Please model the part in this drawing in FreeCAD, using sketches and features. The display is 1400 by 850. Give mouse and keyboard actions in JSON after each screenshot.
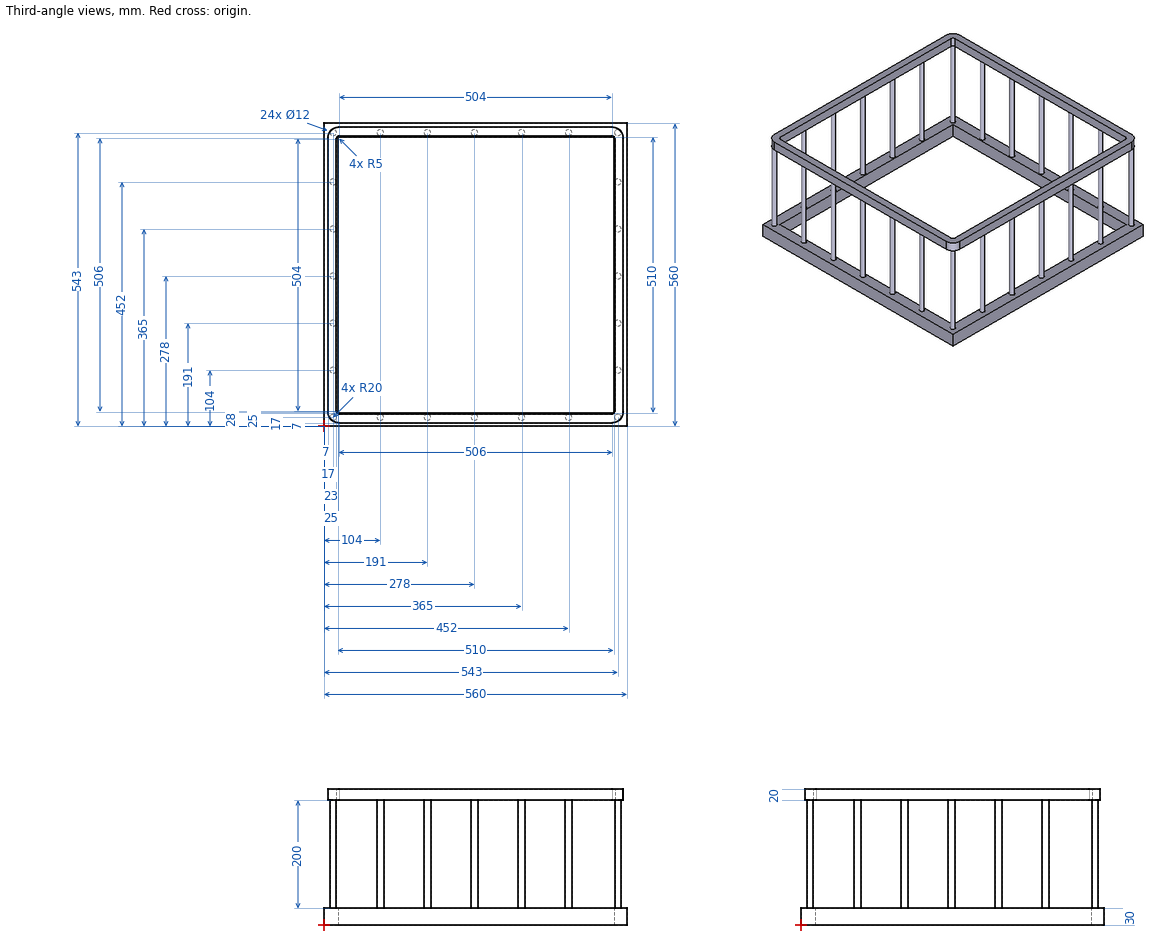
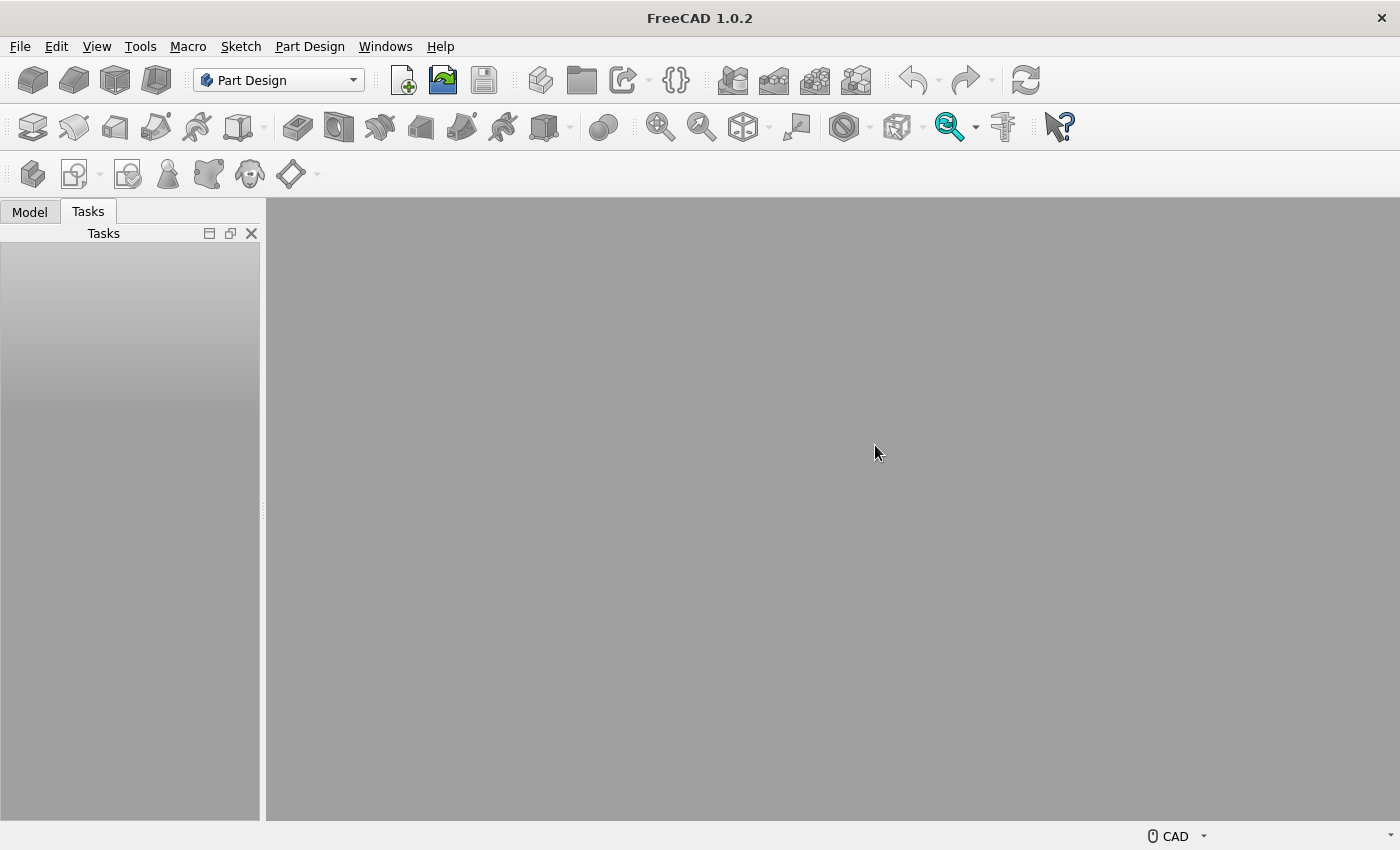
{"action": "left_click", "coordinate": [402, 80]}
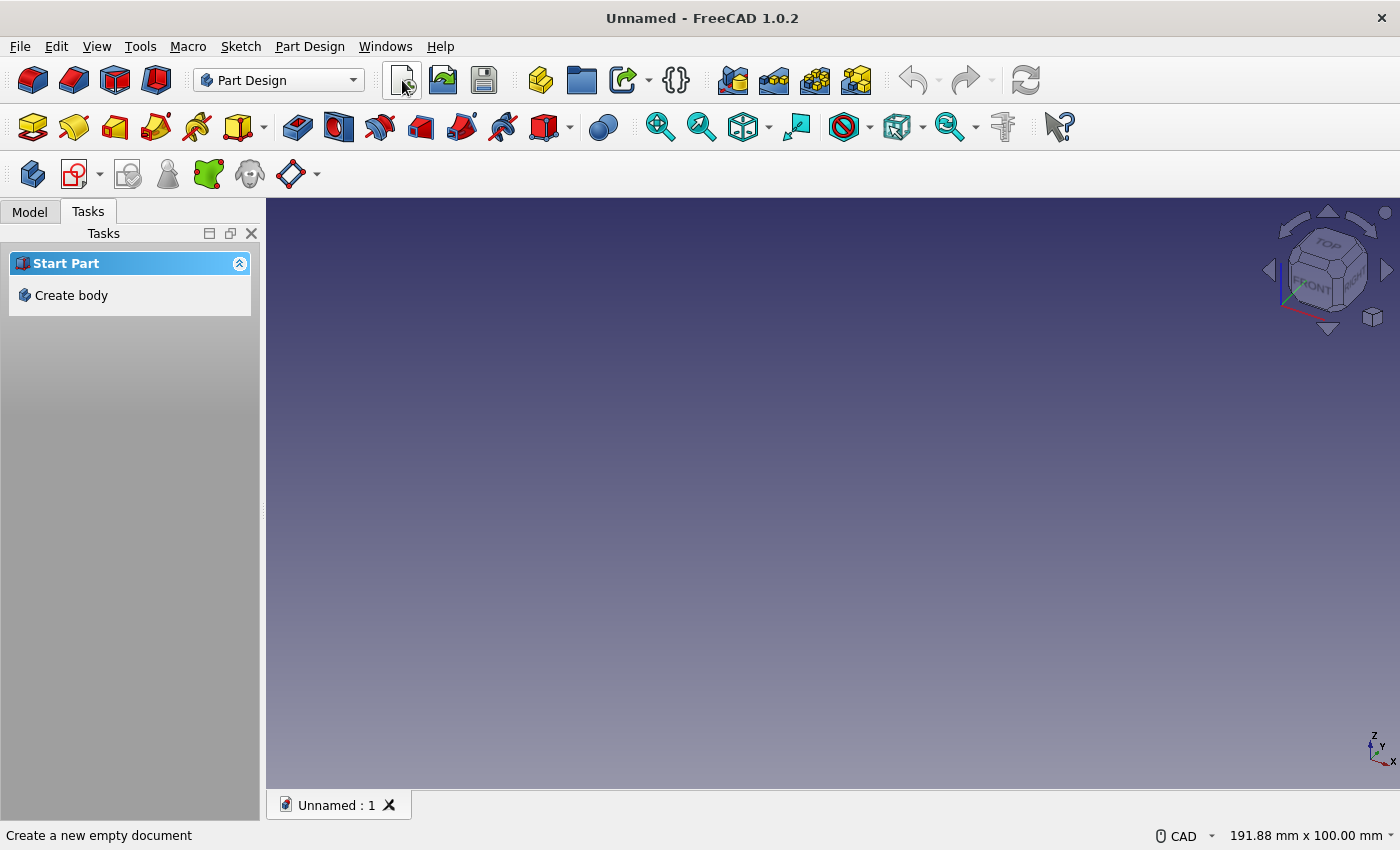
{"action": "left_click", "coordinate": [74, 174]}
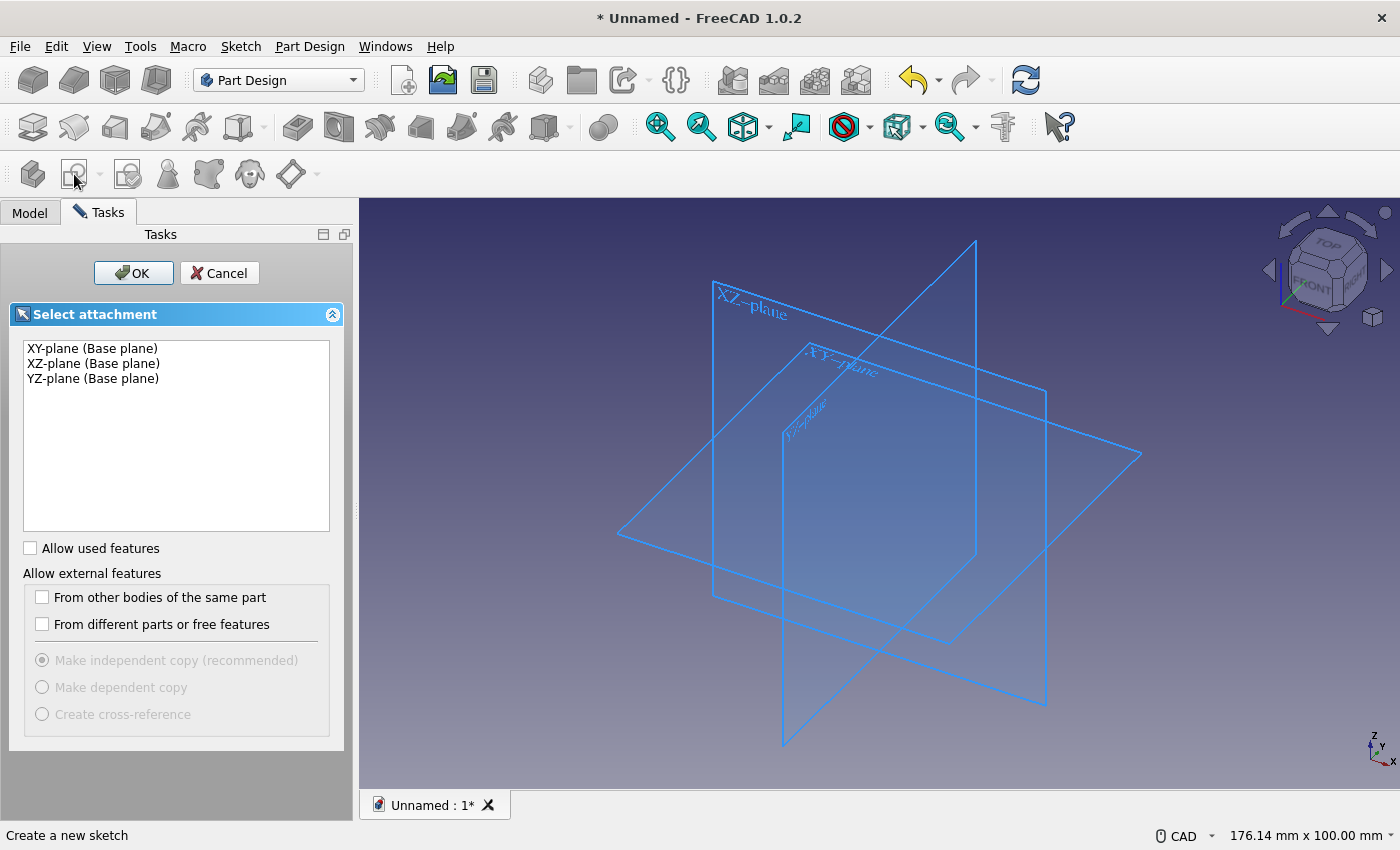
{"action": "left_click", "coordinate": [84, 348]}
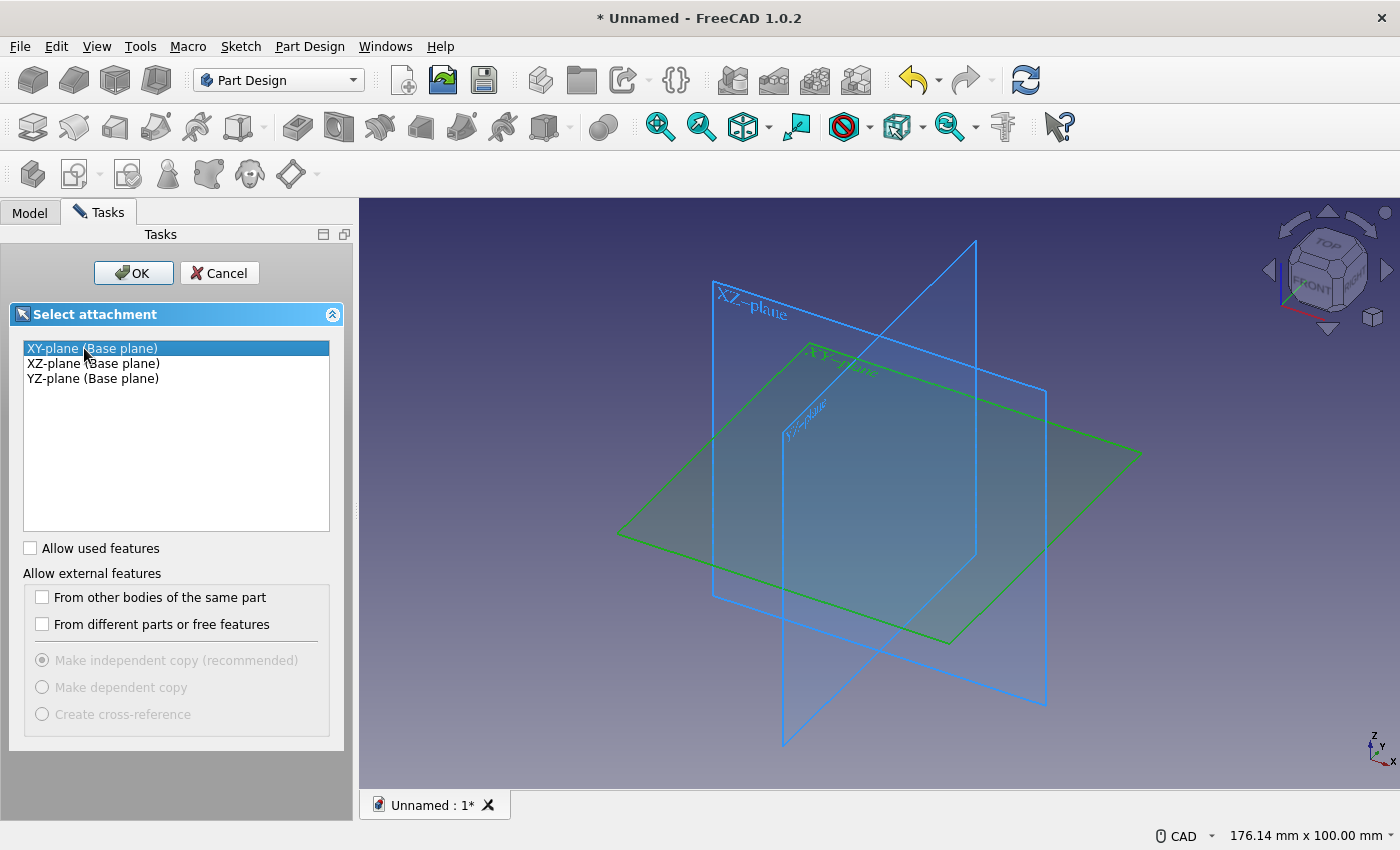
{"action": "left_click", "coordinate": [134, 273]}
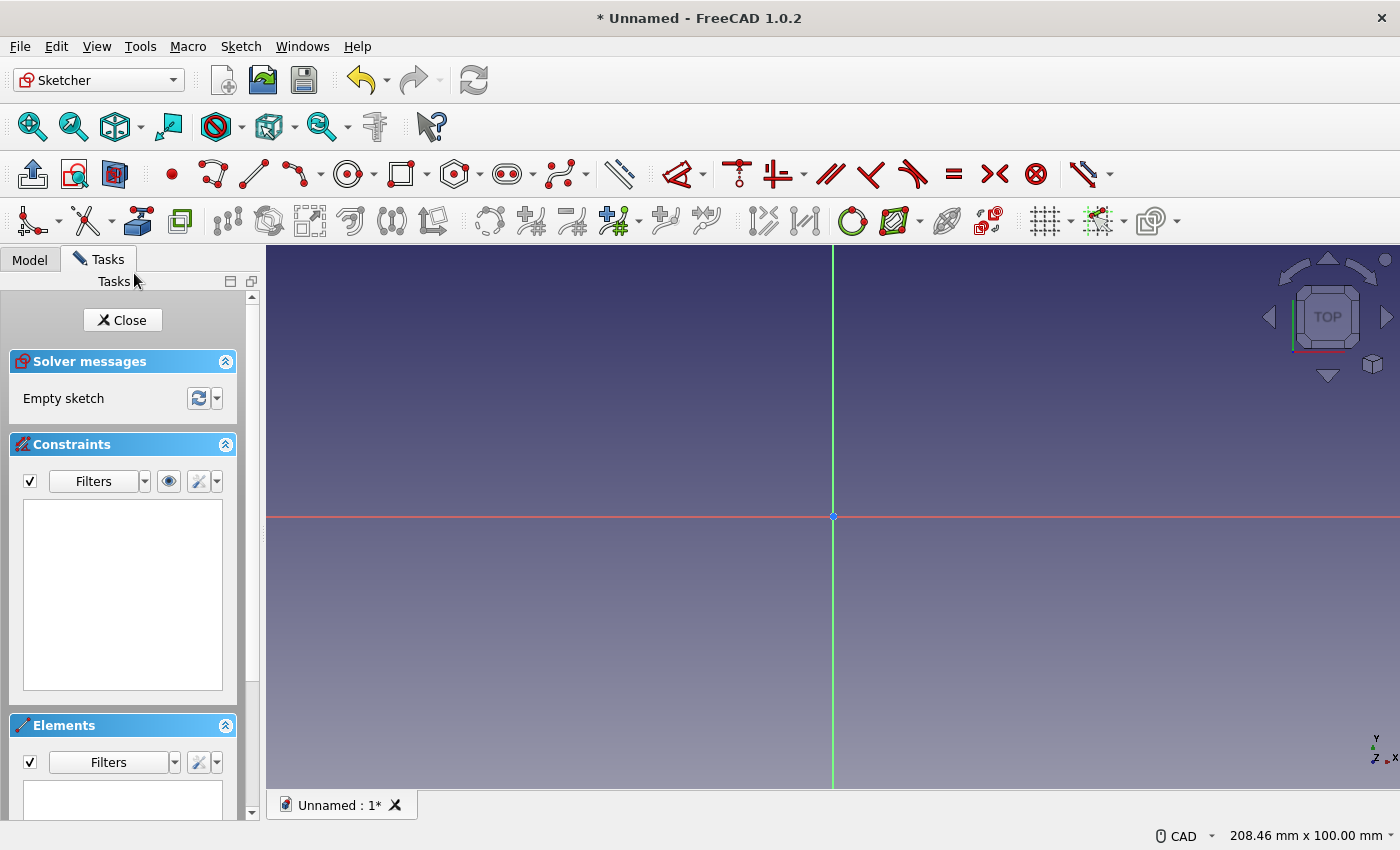
{"action": "scroll", "coordinate": [566, 707], "scroll_direction": "down", "scroll_amount": 11}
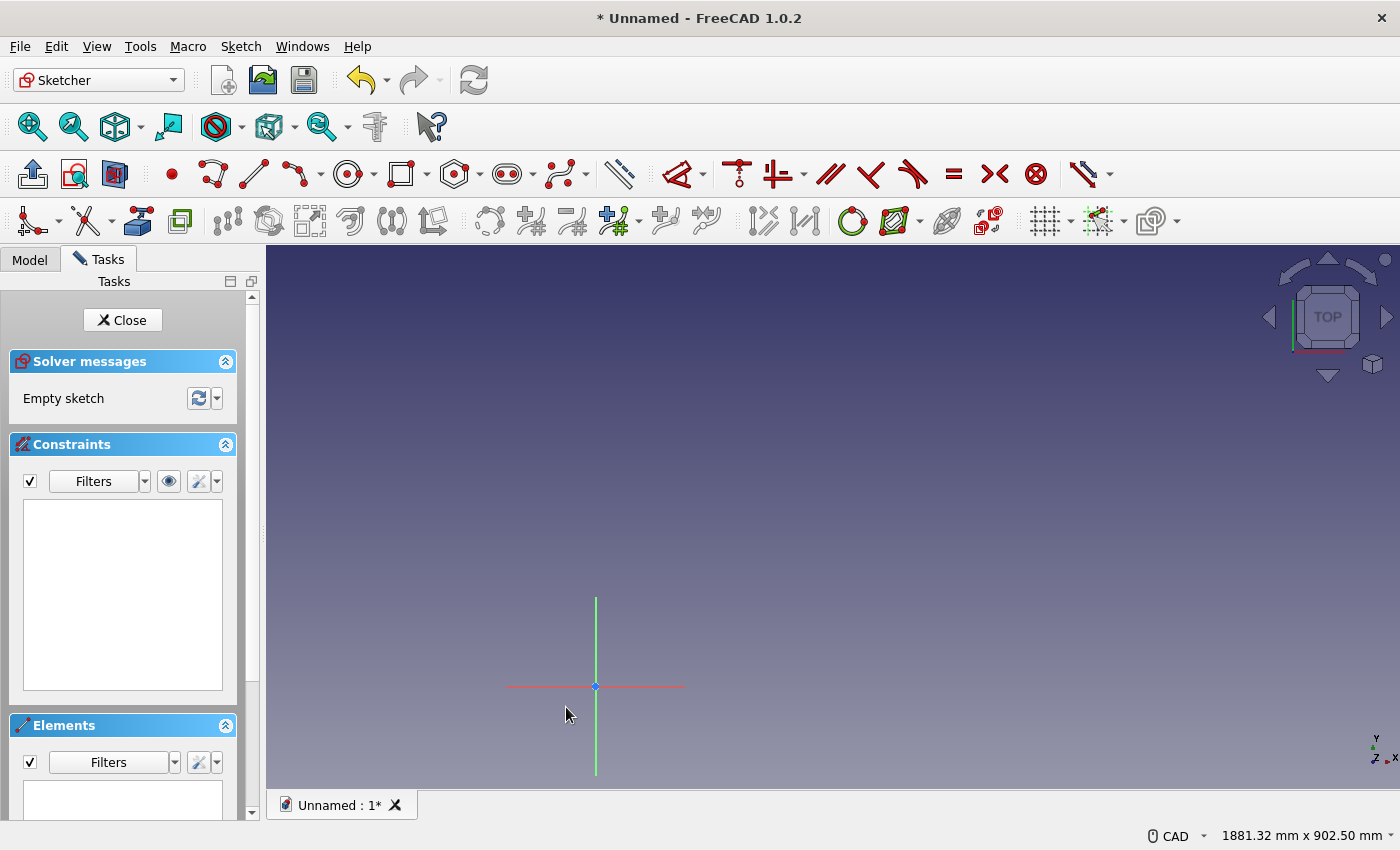
{"action": "left_click", "coordinate": [400, 174]}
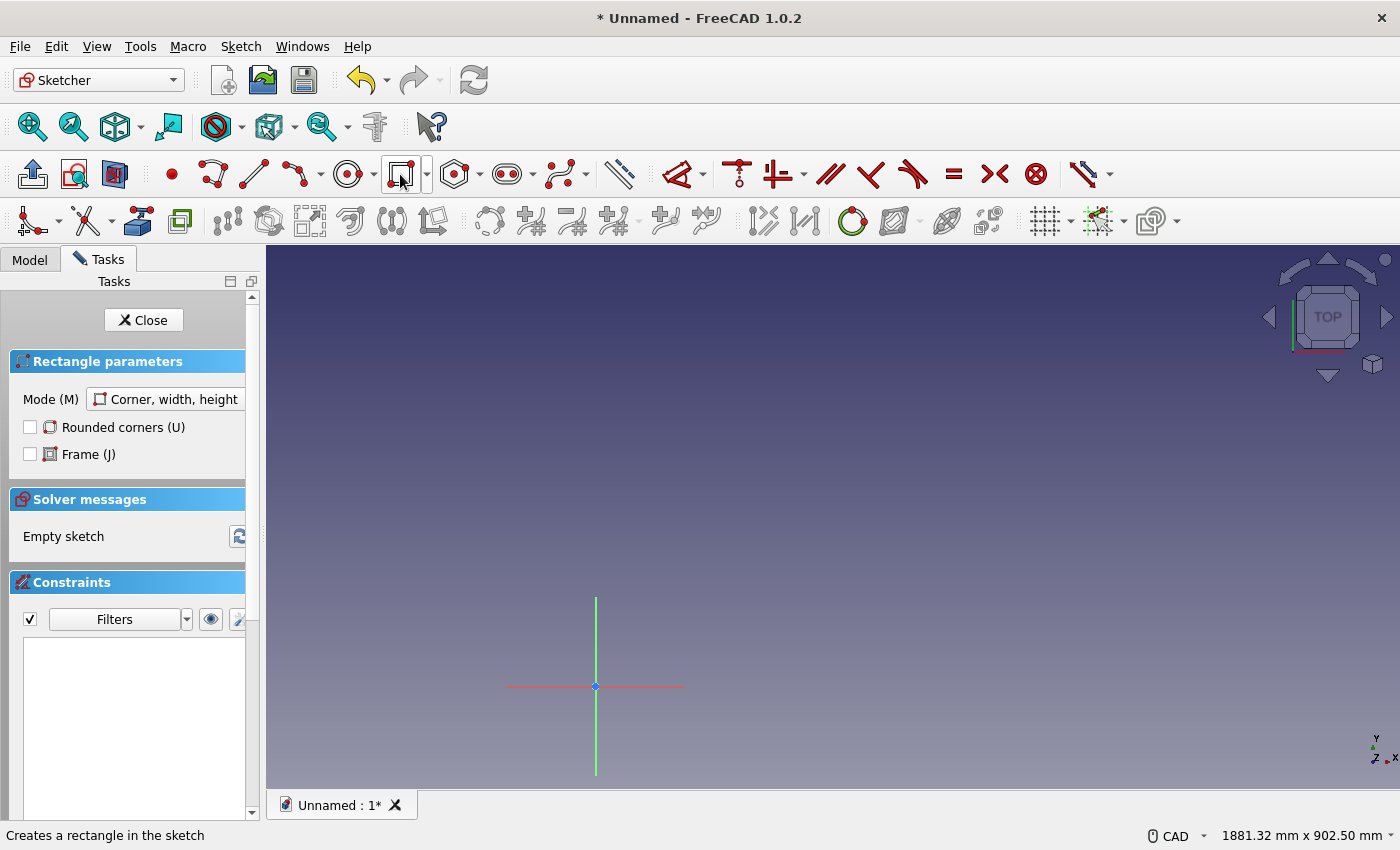
{"action": "left_click", "coordinate": [596, 687]}
{"action": "mouse_move", "coordinate": [933, 349]}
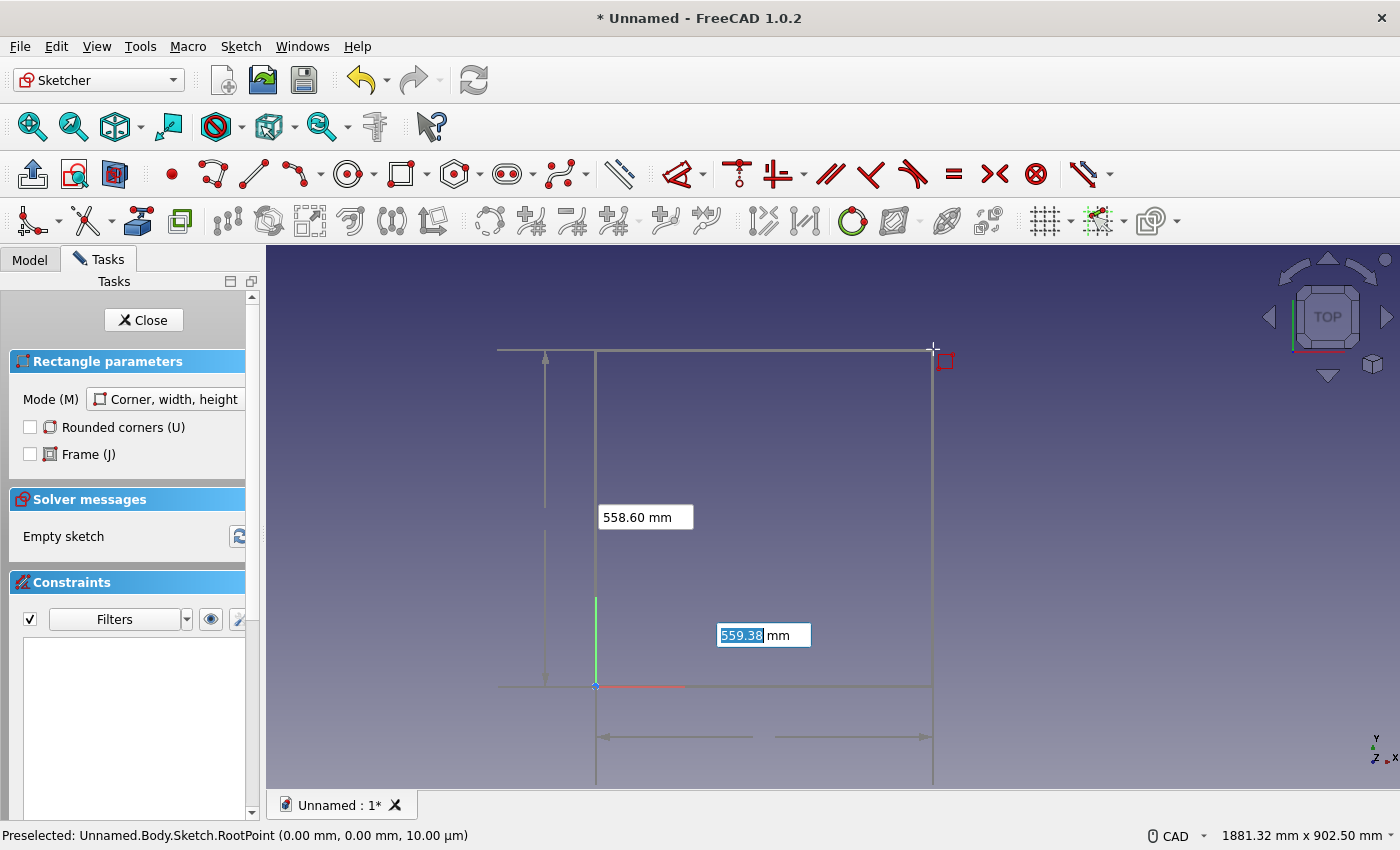
{"action": "type", "text": "560"}
{"action": "key", "text": "Tab"}
{"action": "type", "text": "560"}
{"action": "key", "text": "Return"}